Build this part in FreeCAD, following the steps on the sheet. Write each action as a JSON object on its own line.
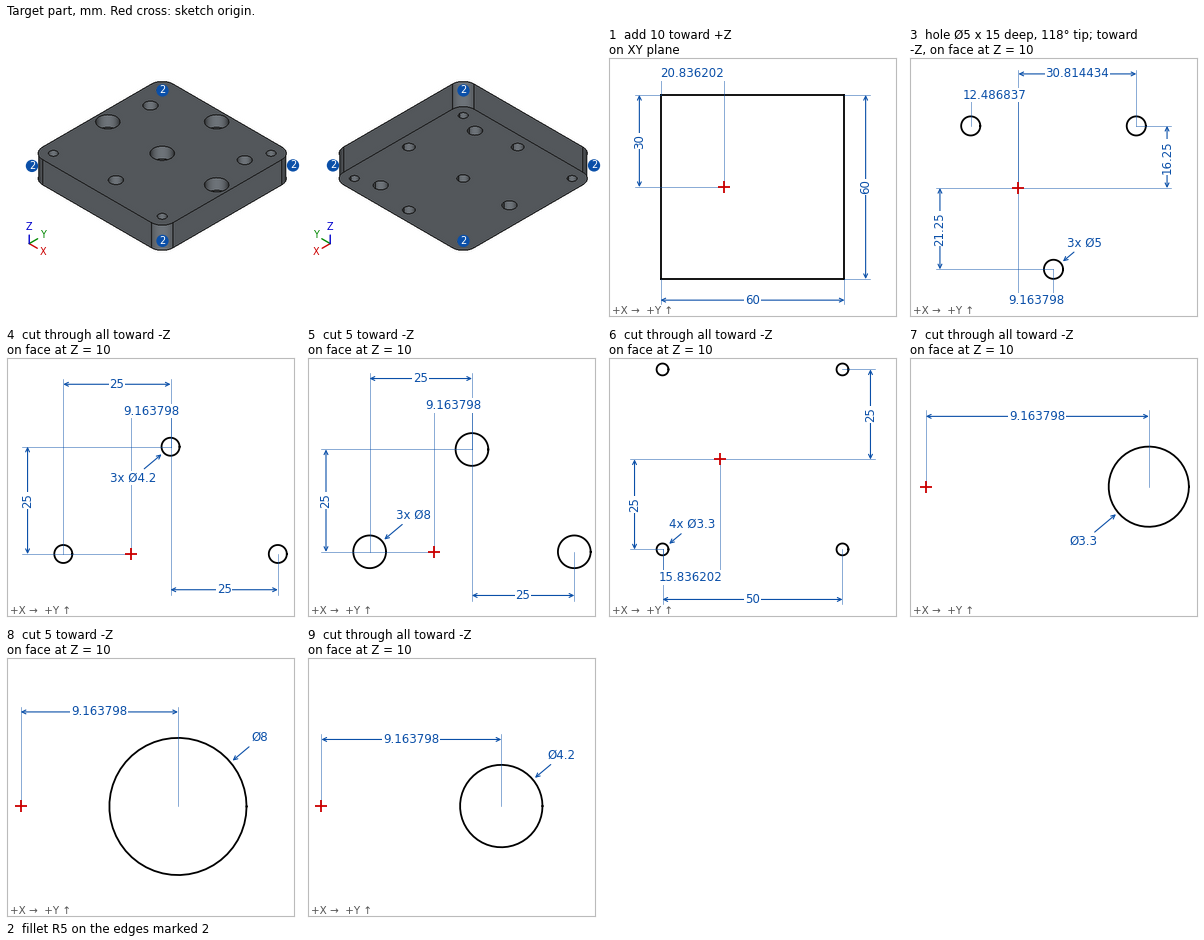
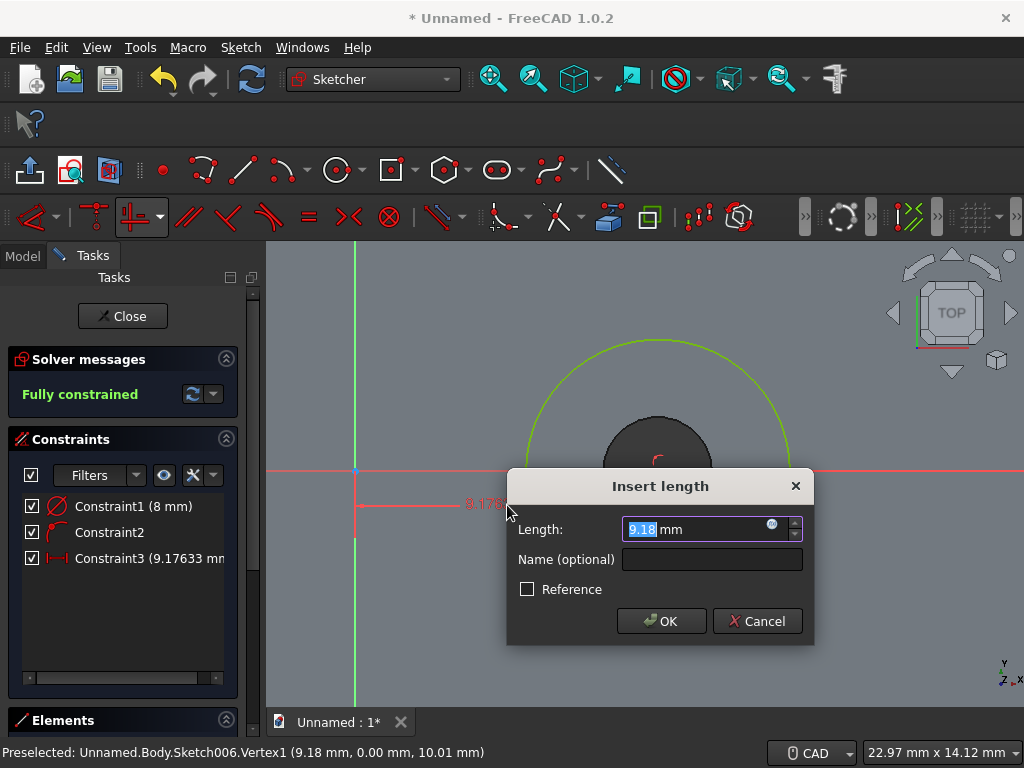
{"action": "type", "text": "9.163798"}
{"action": "key", "text": "Return"}
{"action": "key", "text": "Escape"}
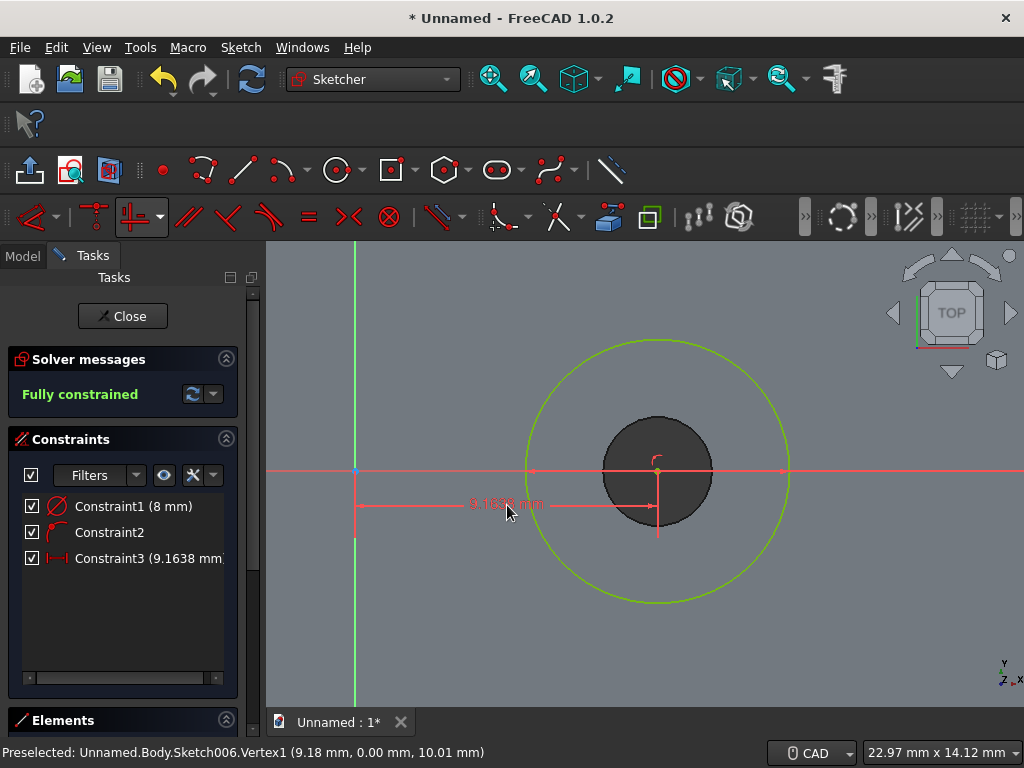
{"action": "left_click", "coordinate": [123, 316]}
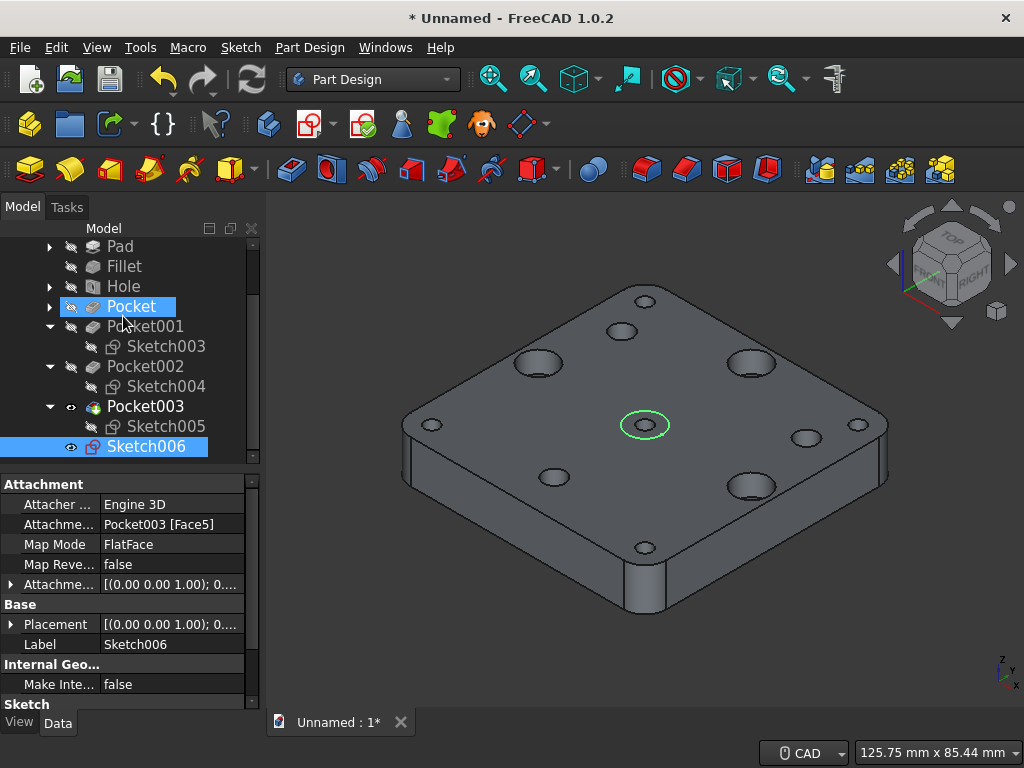
{"action": "left_click", "coordinate": [292, 170]}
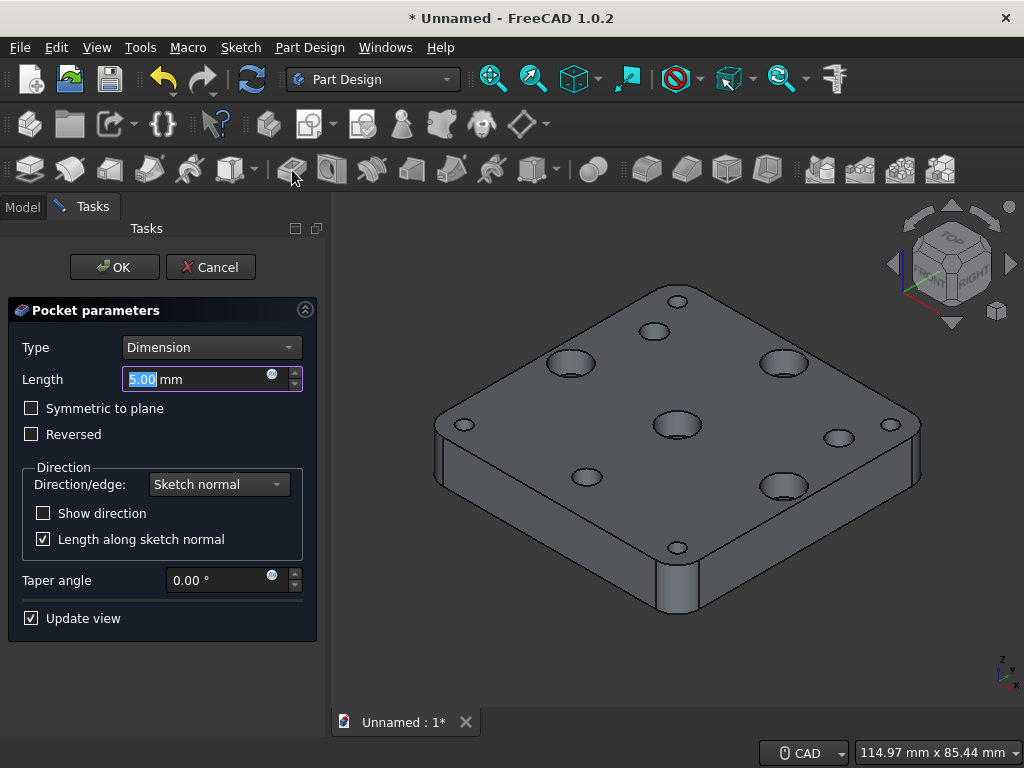
{"action": "type", "text": "5"}
{"action": "key", "text": "Tab"}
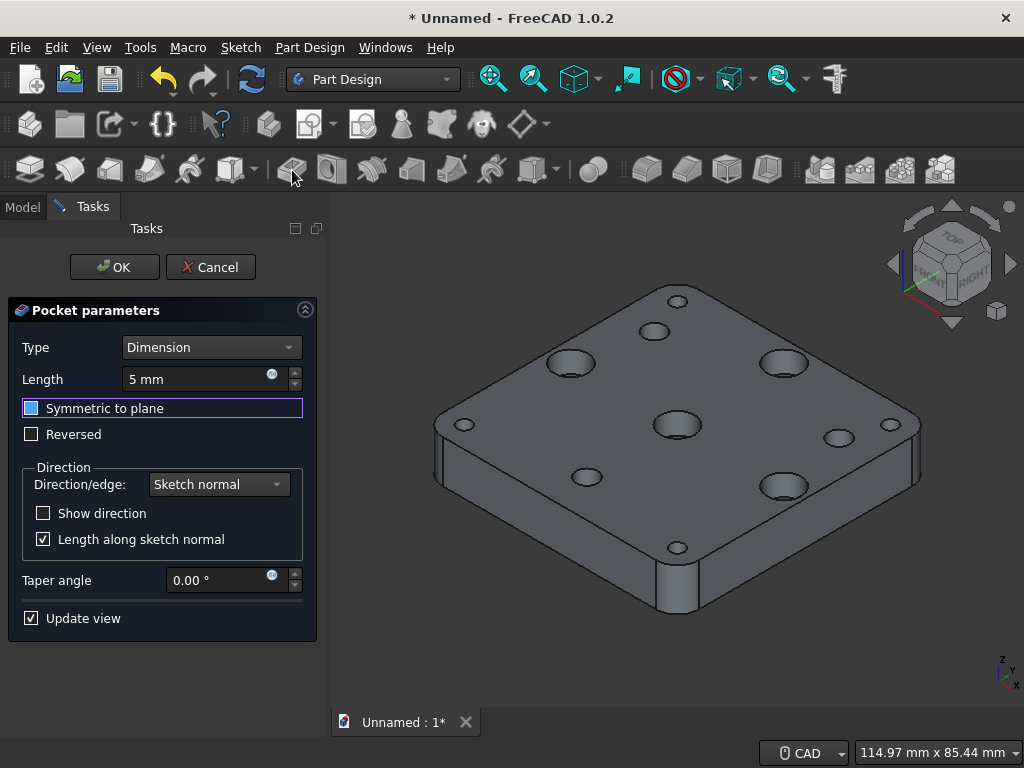
{"action": "left_click", "coordinate": [115, 267]}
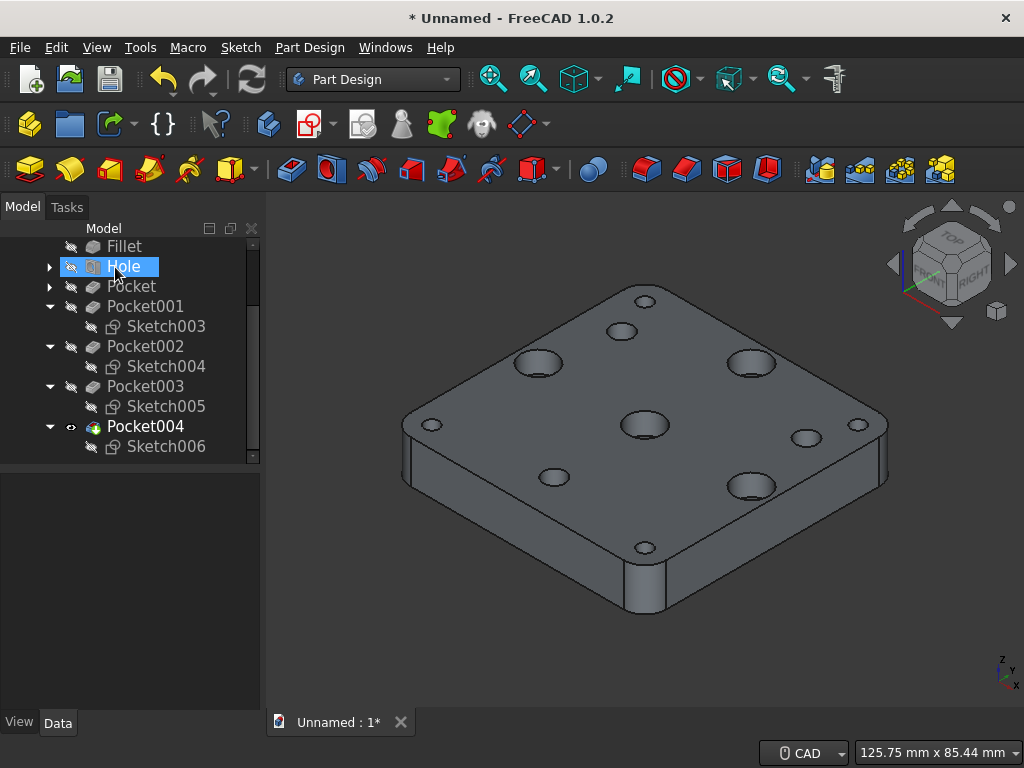
{"action": "left_click", "coordinate": [499, 424]}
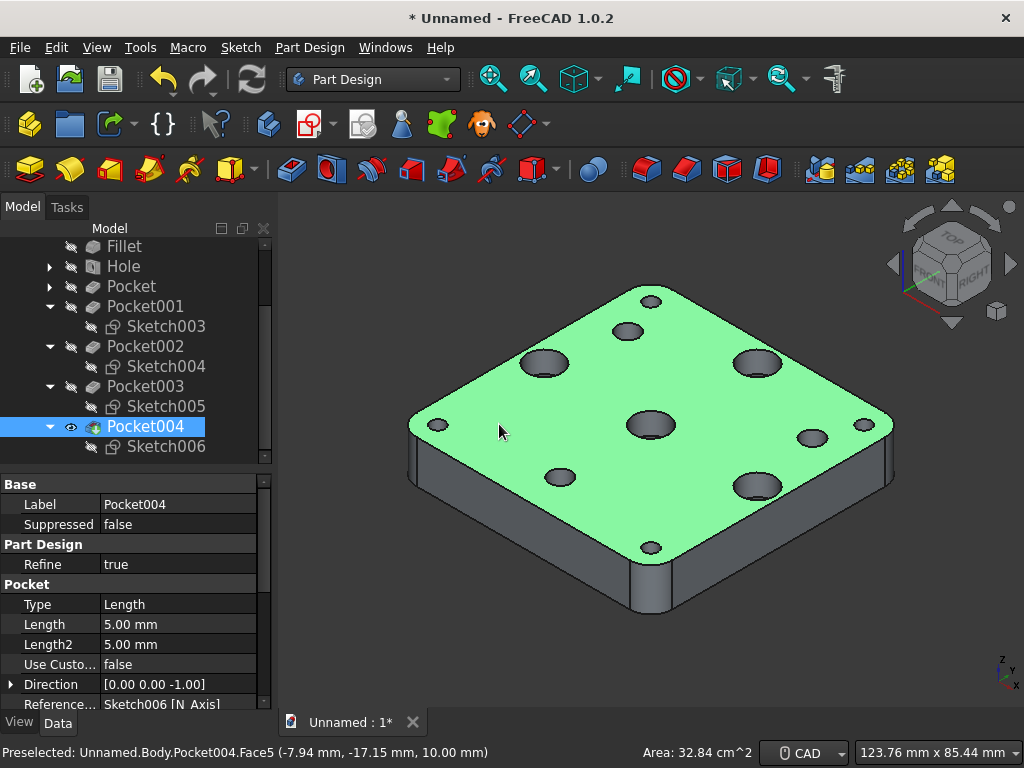
{"action": "left_click", "coordinate": [310, 124]}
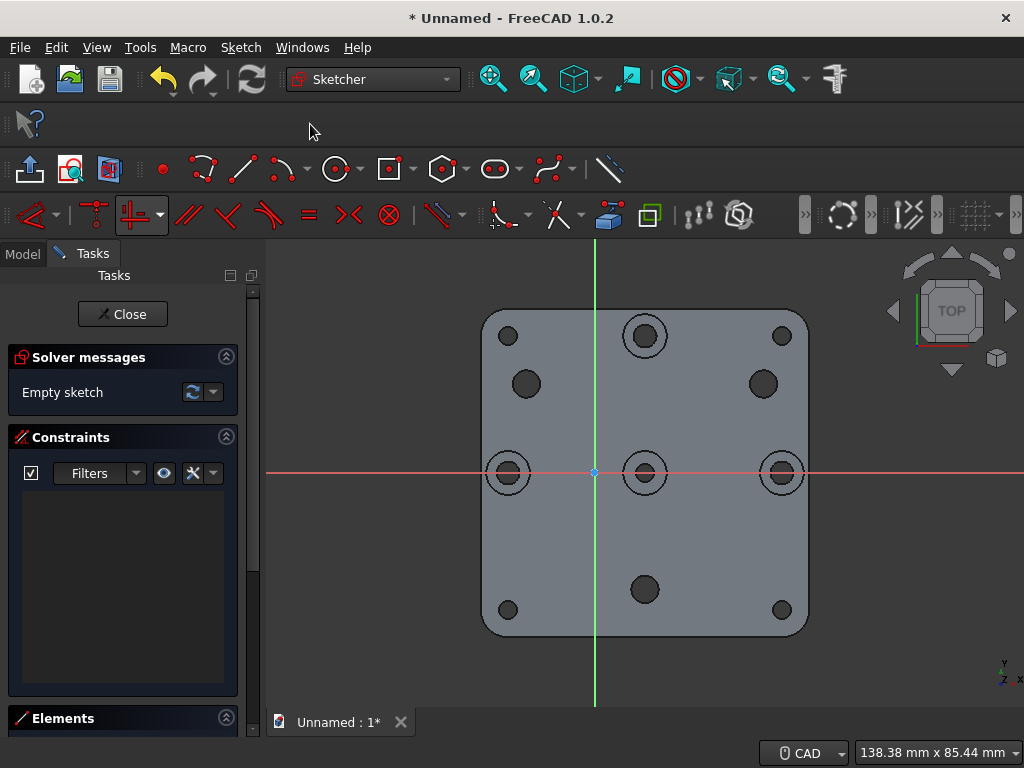
{"action": "scroll", "coordinate": [650, 473], "scroll_direction": "up", "scroll_amount": 13}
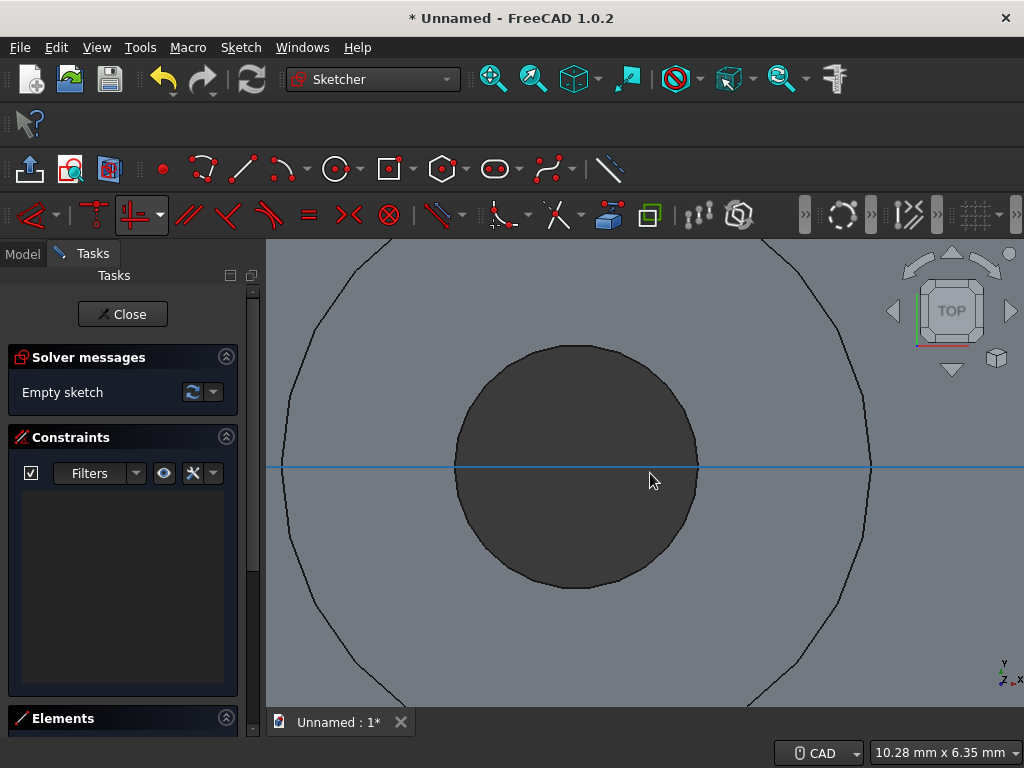
{"action": "left_click", "coordinate": [336, 170]}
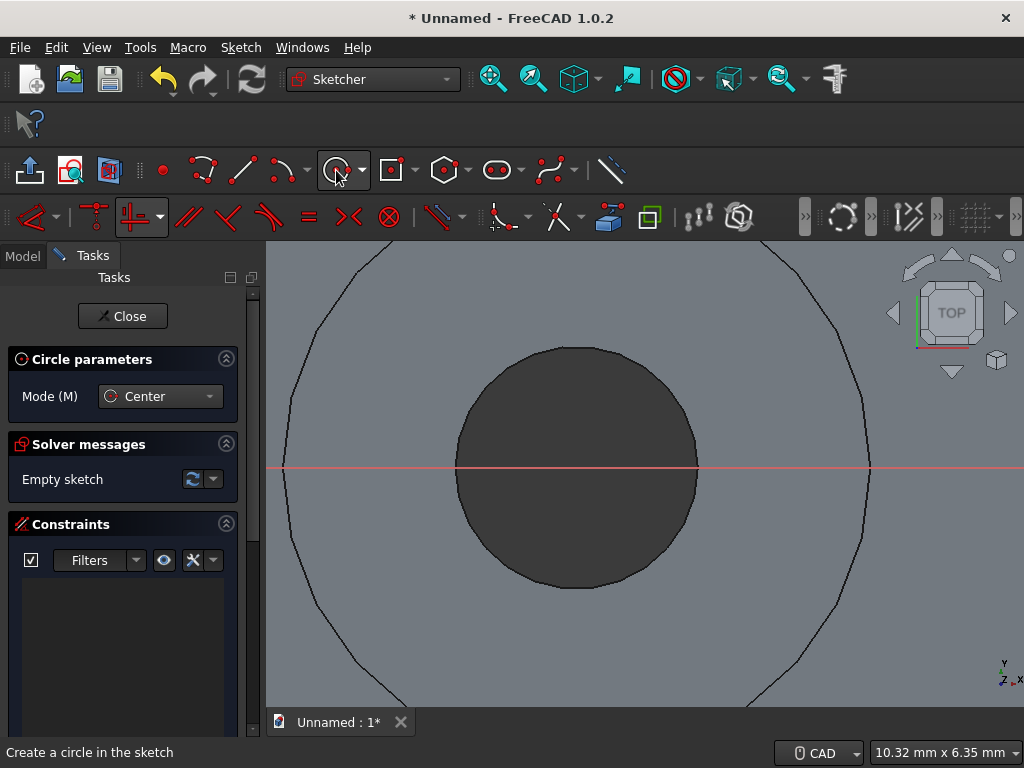
{"action": "left_click", "coordinate": [577, 468]}
{"action": "mouse_move", "coordinate": [686, 359]}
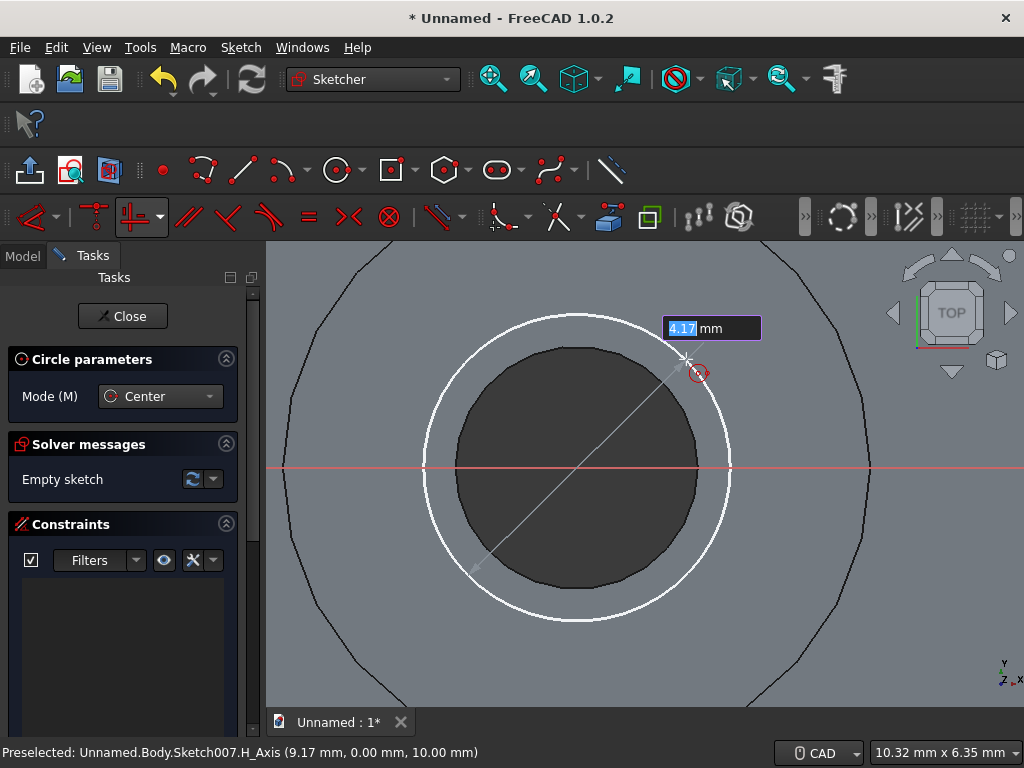
{"action": "type", "text": "4.2"}
{"action": "key", "text": "Return"}
{"action": "key", "text": "Escape"}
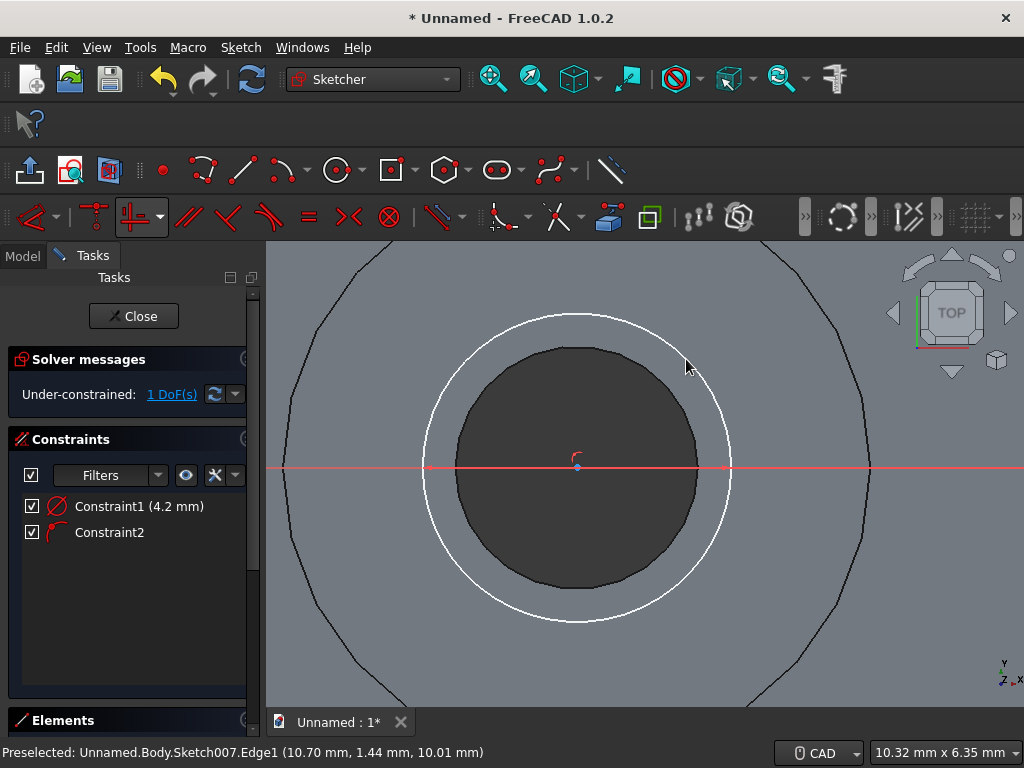
{"action": "left_click", "coordinate": [32, 218]}